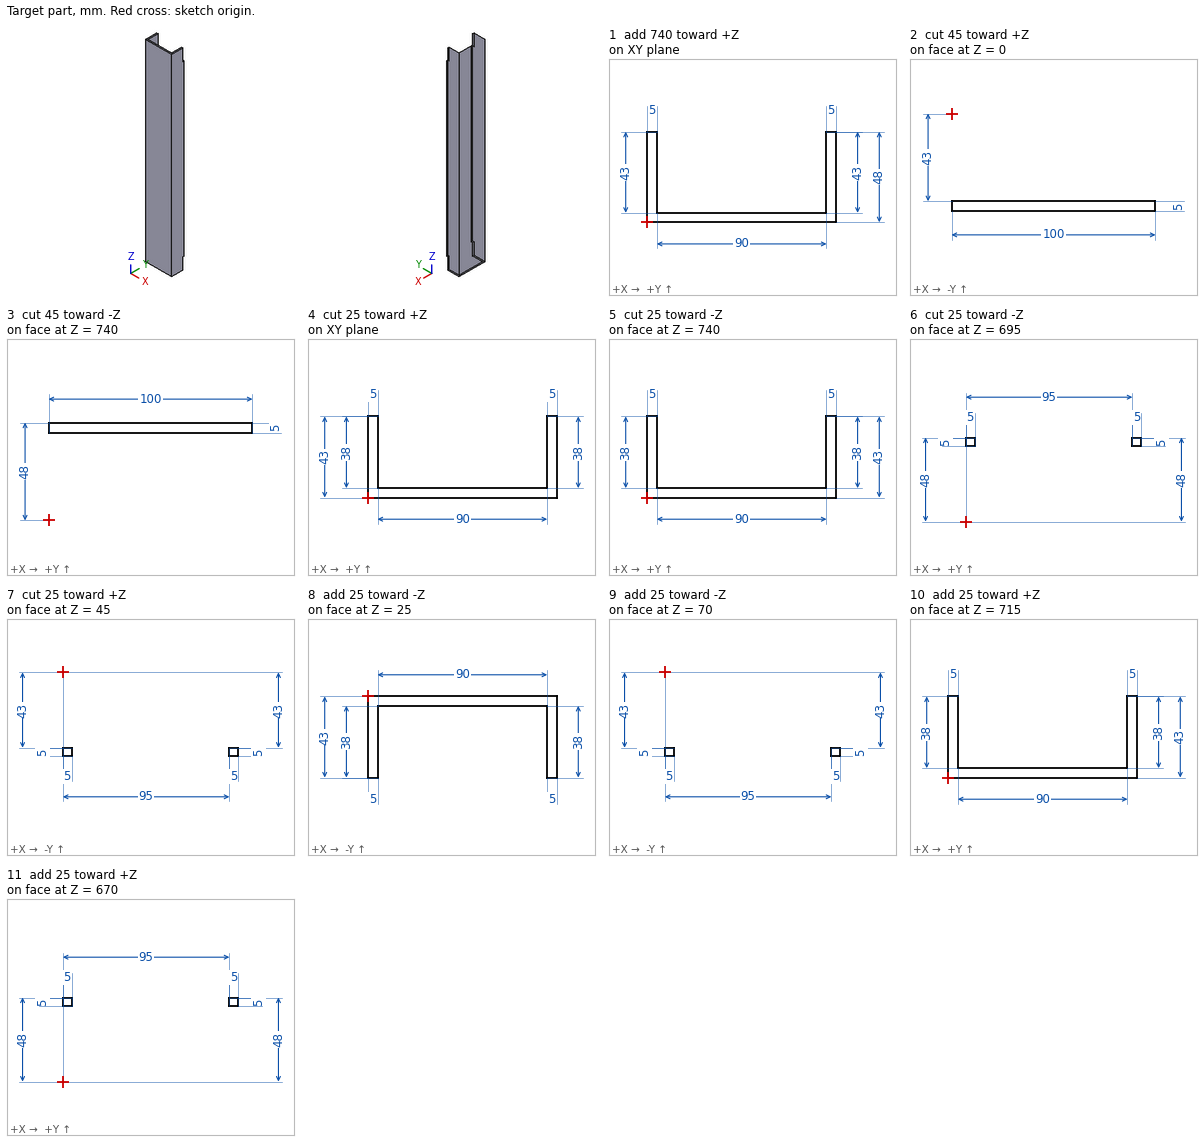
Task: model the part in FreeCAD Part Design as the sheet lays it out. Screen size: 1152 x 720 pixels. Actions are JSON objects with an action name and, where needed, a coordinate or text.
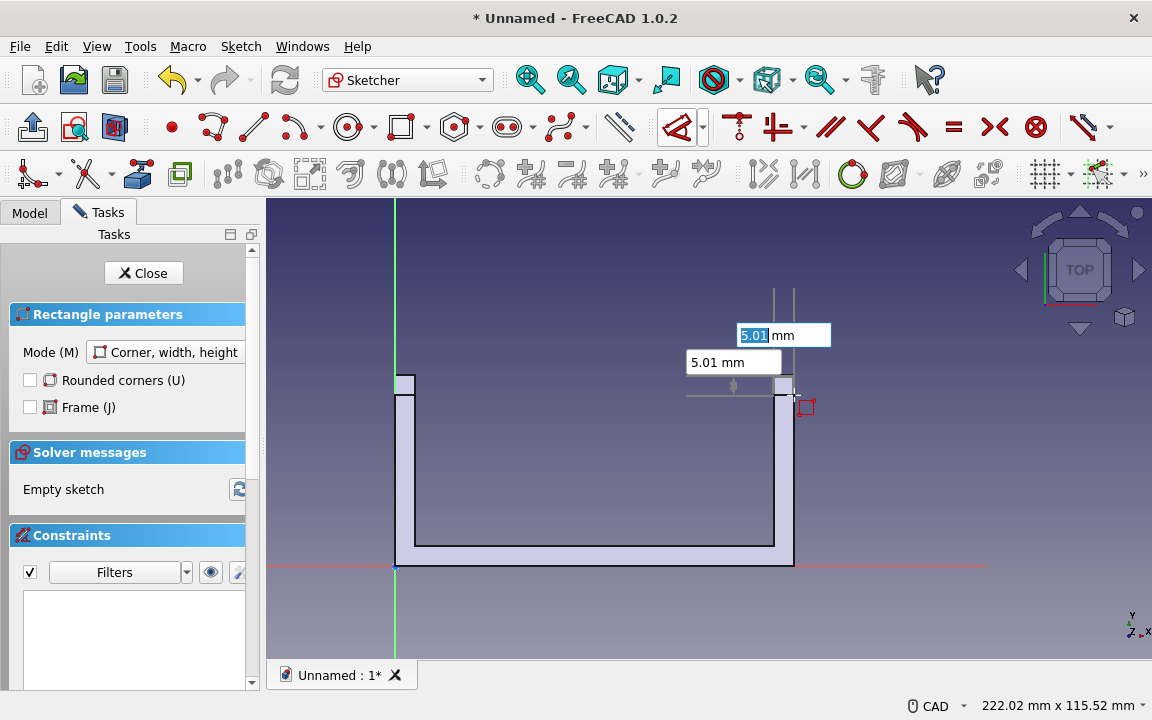
{"action": "type", "text": "5"}
{"action": "key", "text": "Tab"}
{"action": "type", "text": "5"}
{"action": "key", "text": "Return"}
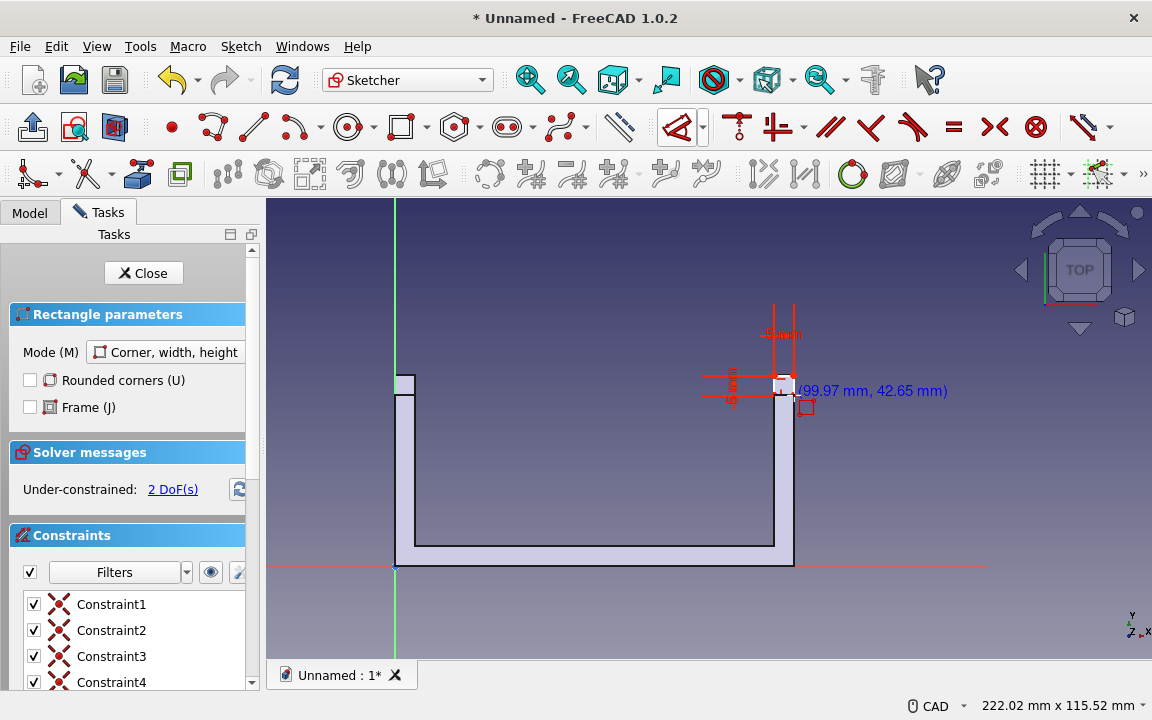
{"action": "left_click", "coordinate": [395, 375]}
{"action": "mouse_move", "coordinate": [415, 395]}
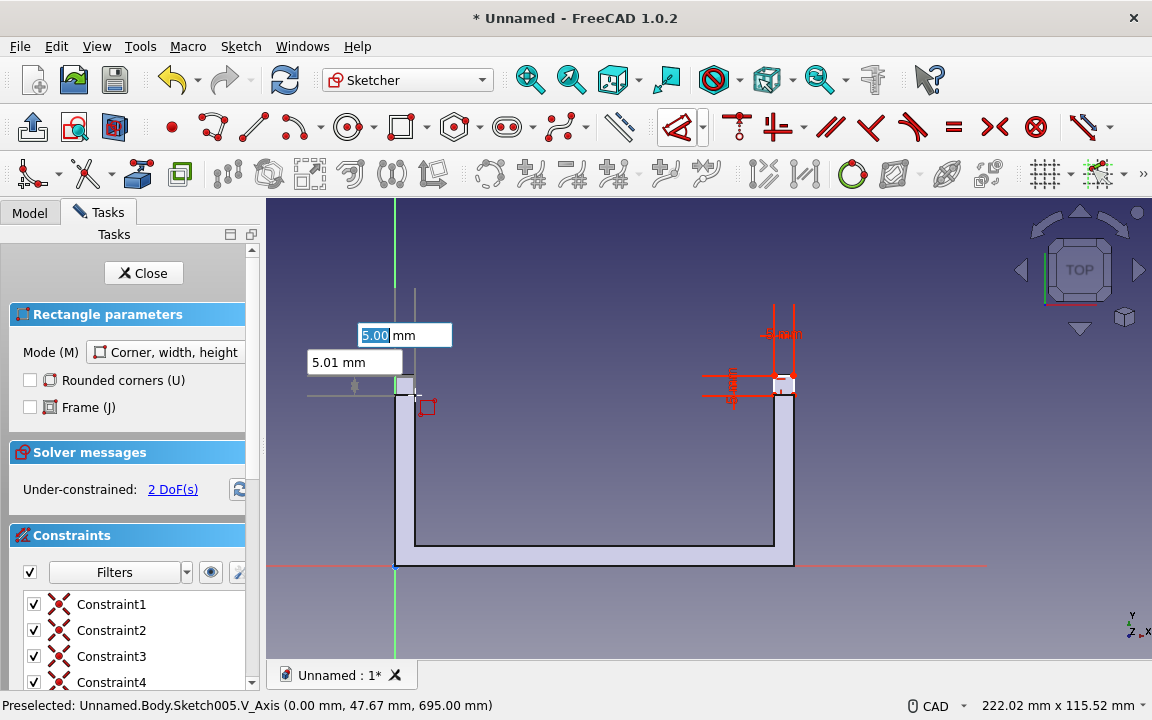
{"action": "type", "text": "5"}
{"action": "key", "text": "Tab"}
{"action": "type", "text": "5"}
{"action": "key", "text": "Return"}
{"action": "key", "text": "Escape"}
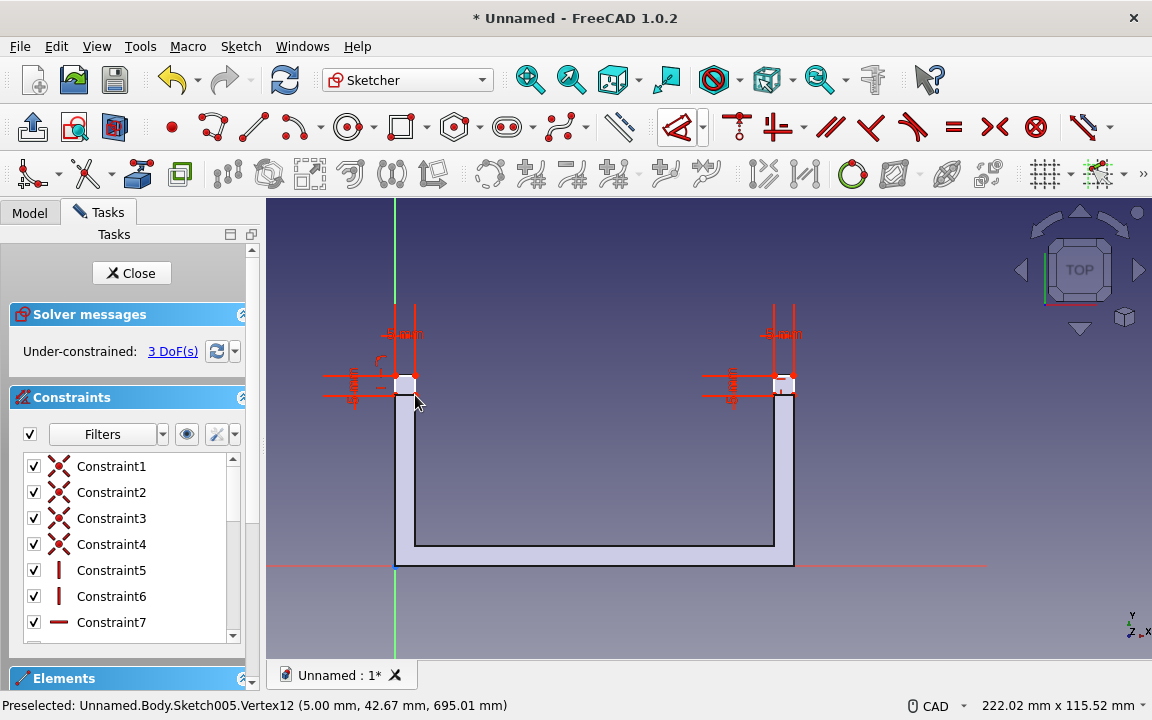
{"action": "left_click", "coordinate": [774, 376]}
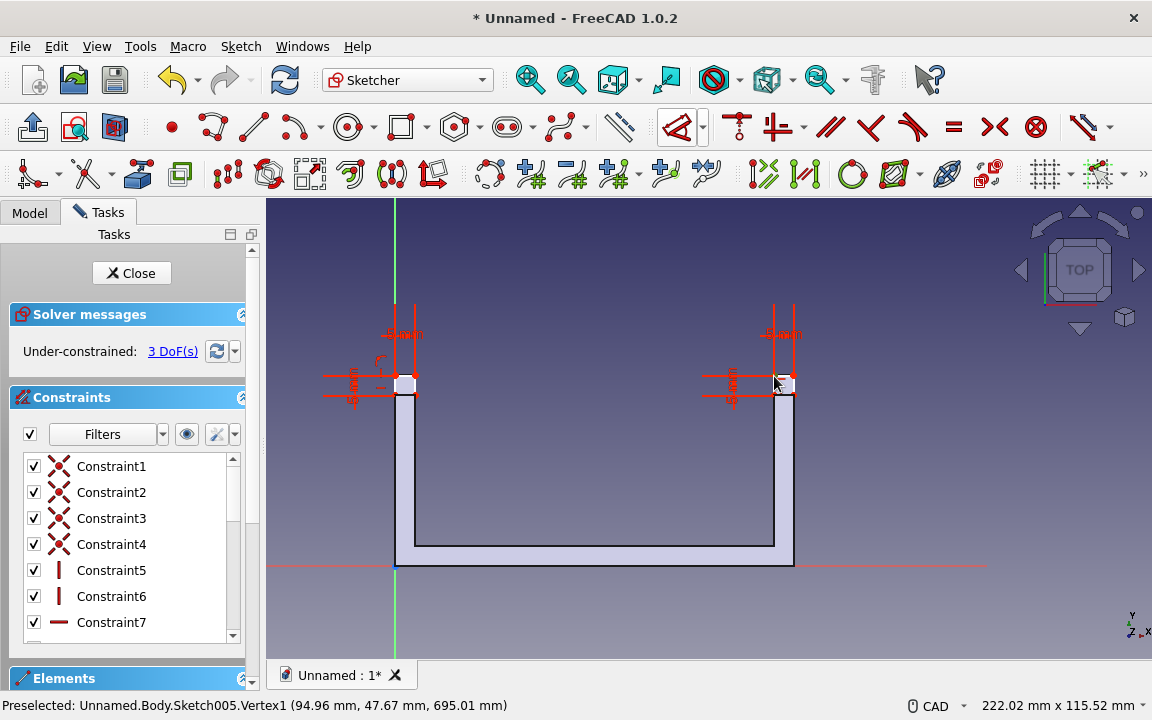
{"action": "left_click", "coordinate": [702, 128]}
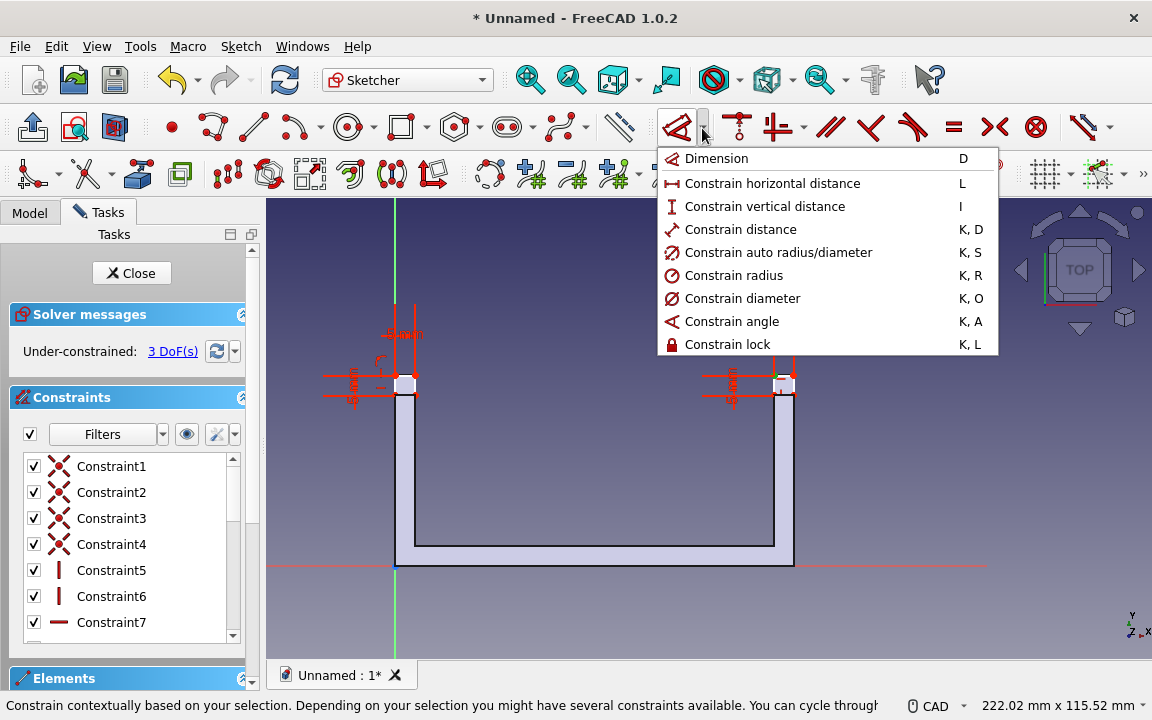
{"action": "left_click", "coordinate": [828, 184]}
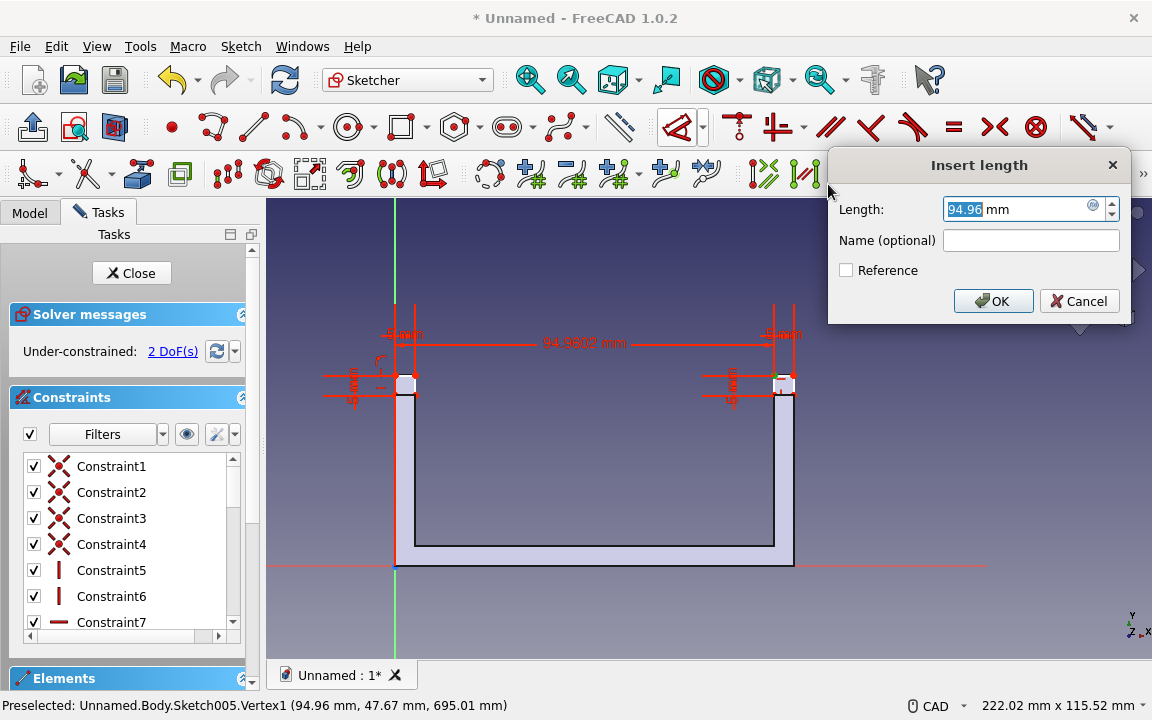
{"action": "type", "text": "95"}
{"action": "key", "text": "Return"}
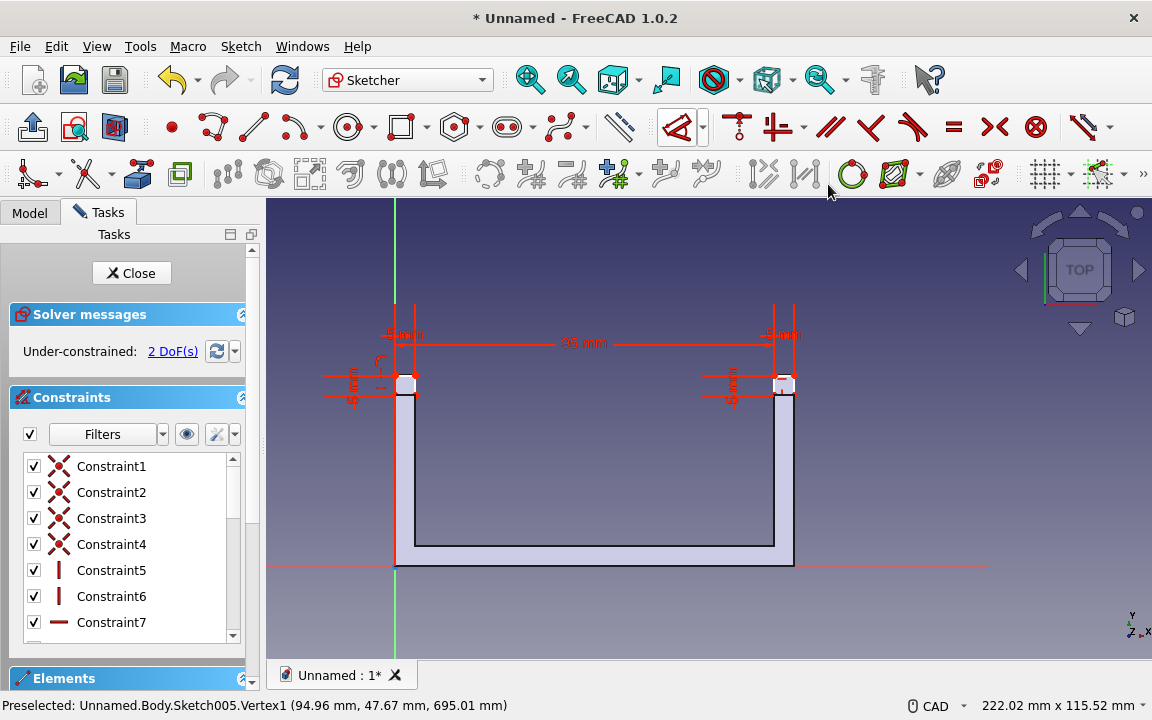
{"action": "left_click", "coordinate": [774, 376]}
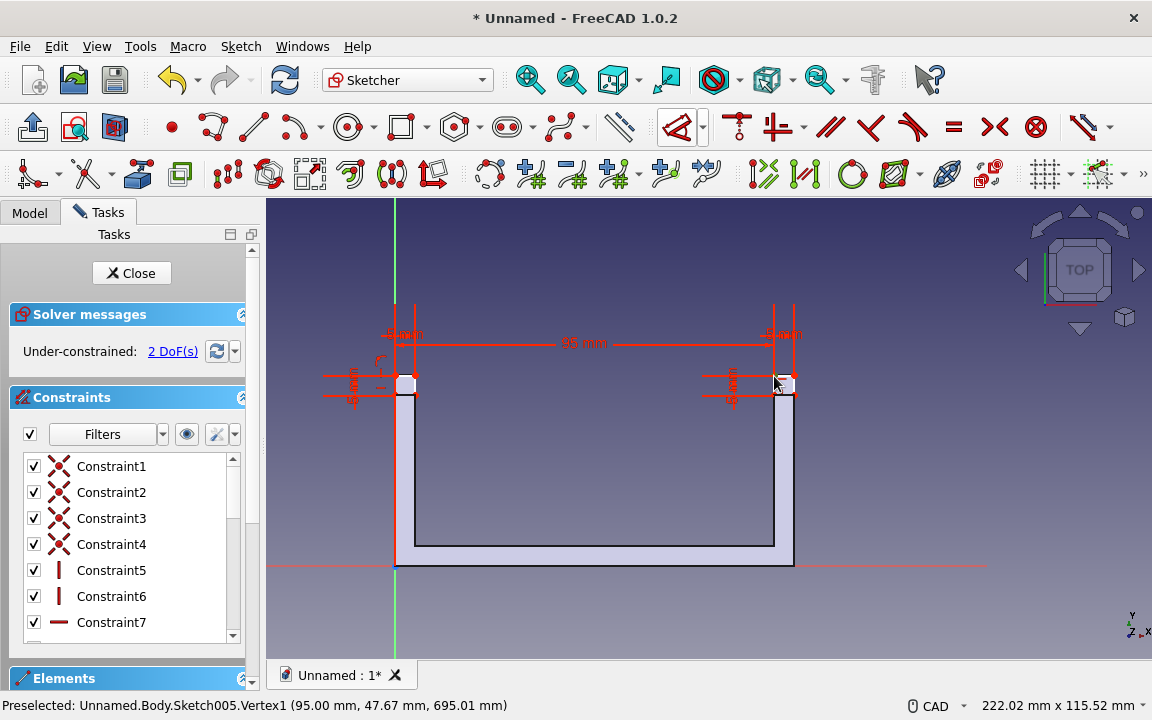
{"action": "key", "text": "i"}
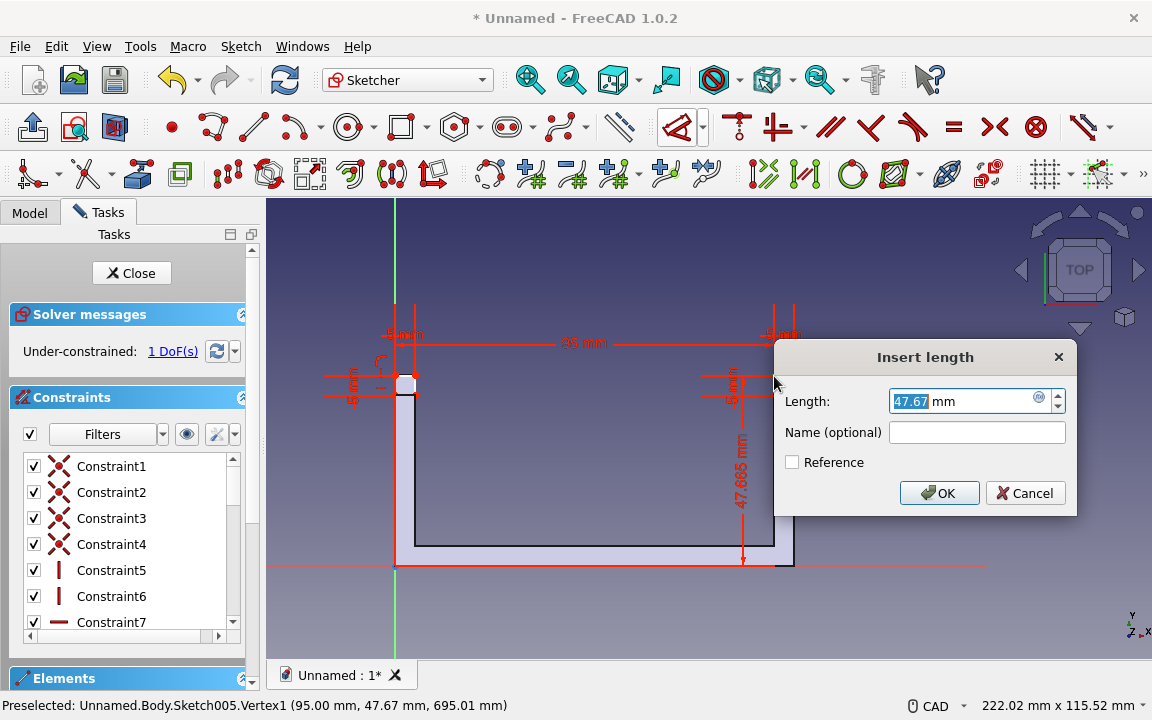
{"action": "type", "text": "48"}
{"action": "key", "text": "Return"}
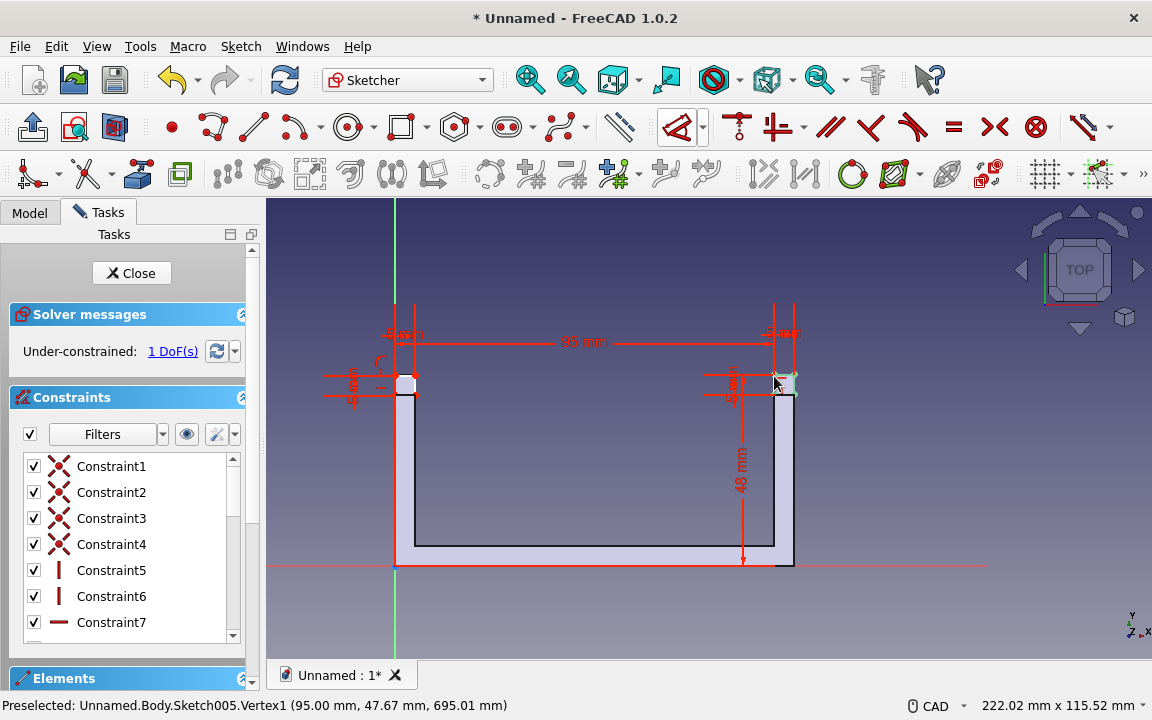
{"action": "left_click", "coordinate": [395, 376]}